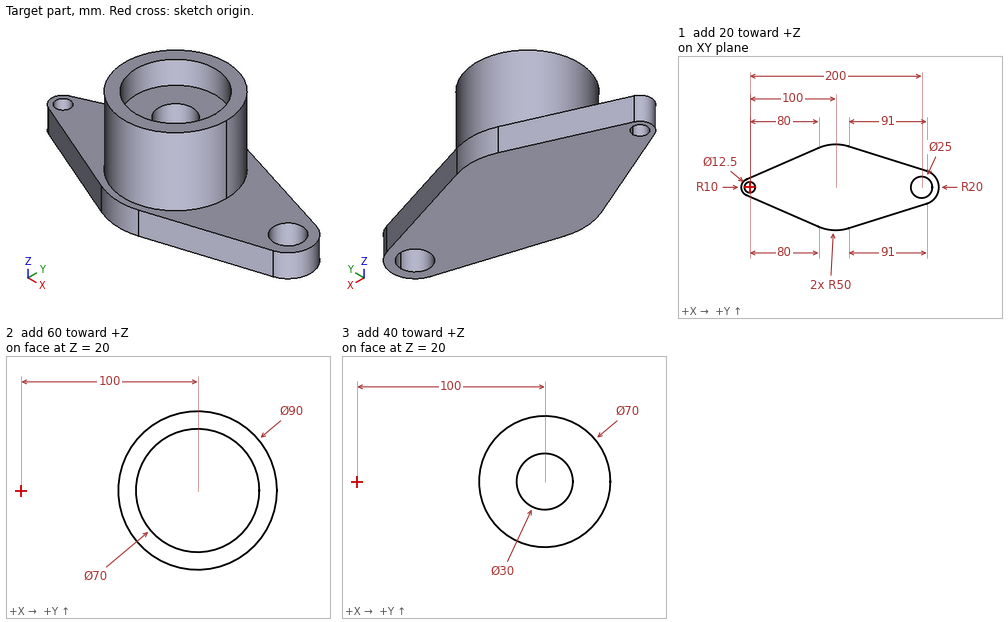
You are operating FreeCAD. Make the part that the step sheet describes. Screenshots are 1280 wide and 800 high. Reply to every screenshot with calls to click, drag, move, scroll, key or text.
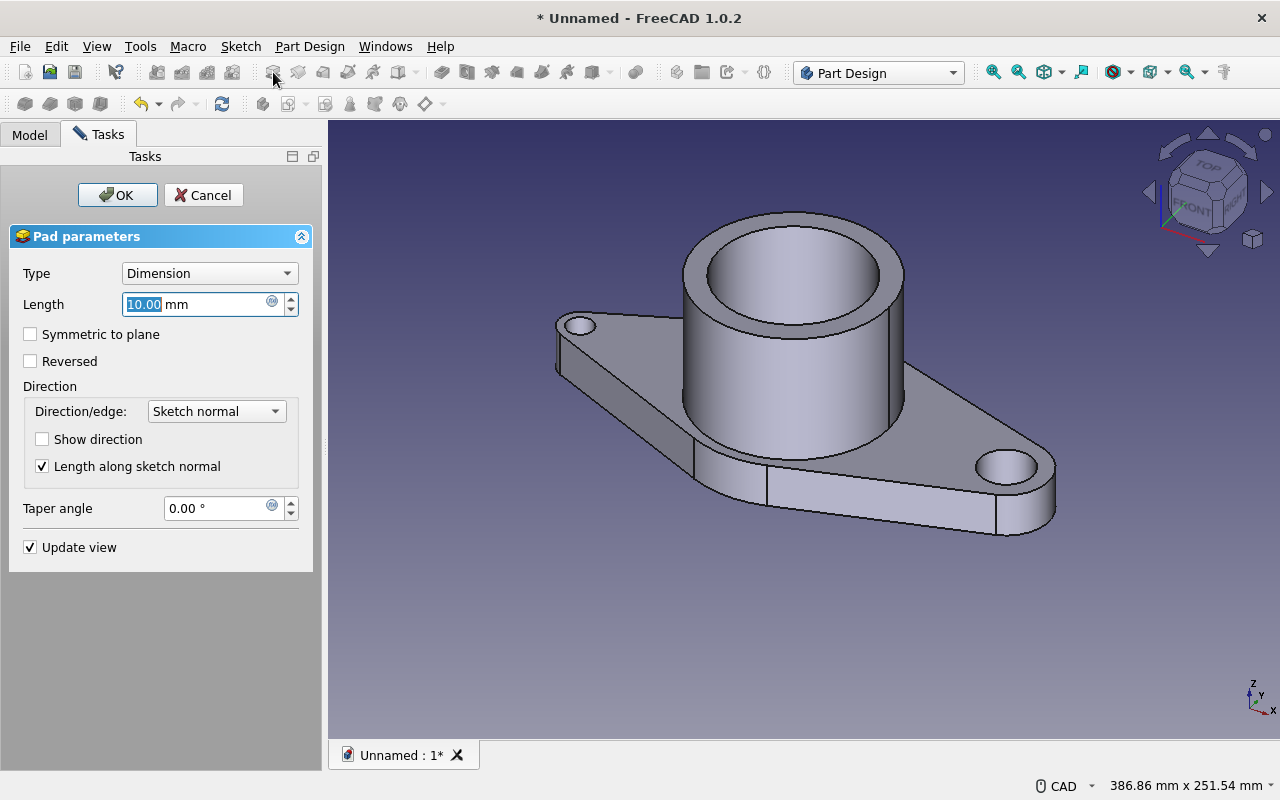
text(40)
key(Tab)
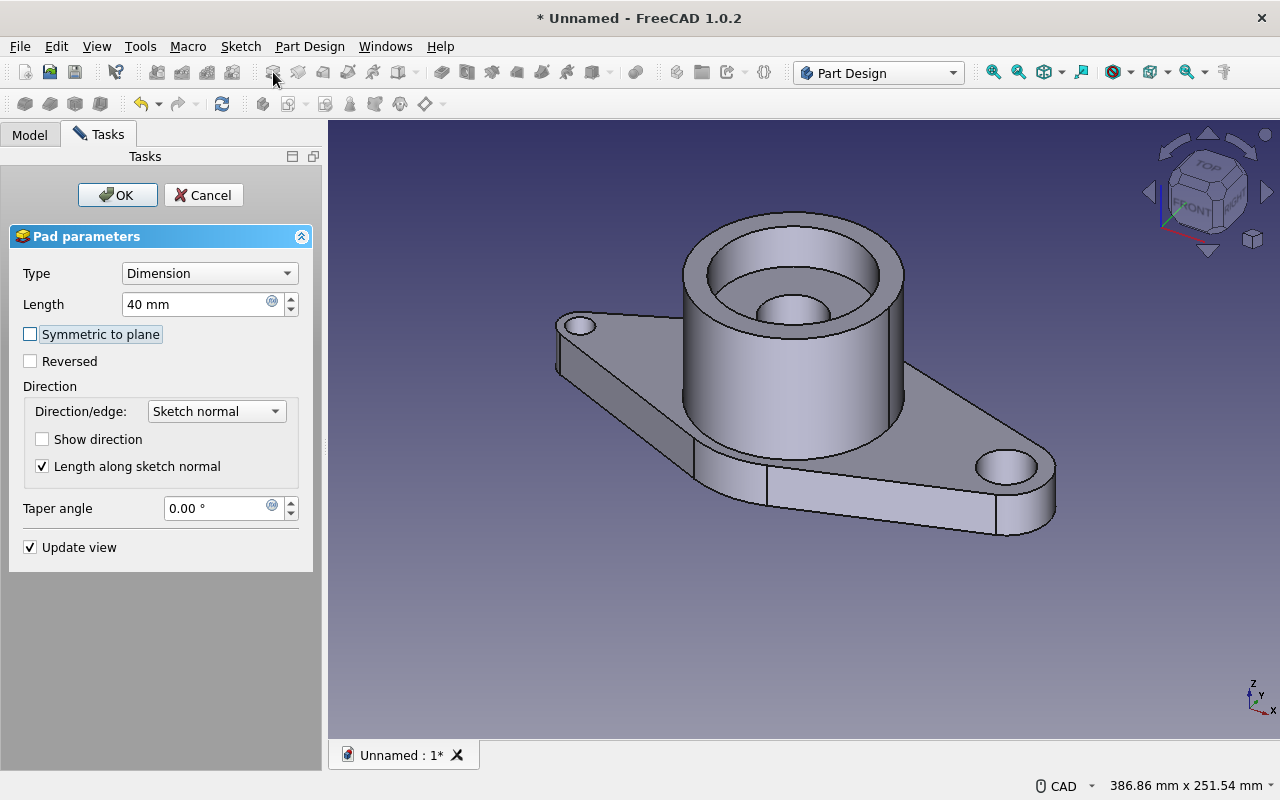
click(118, 195)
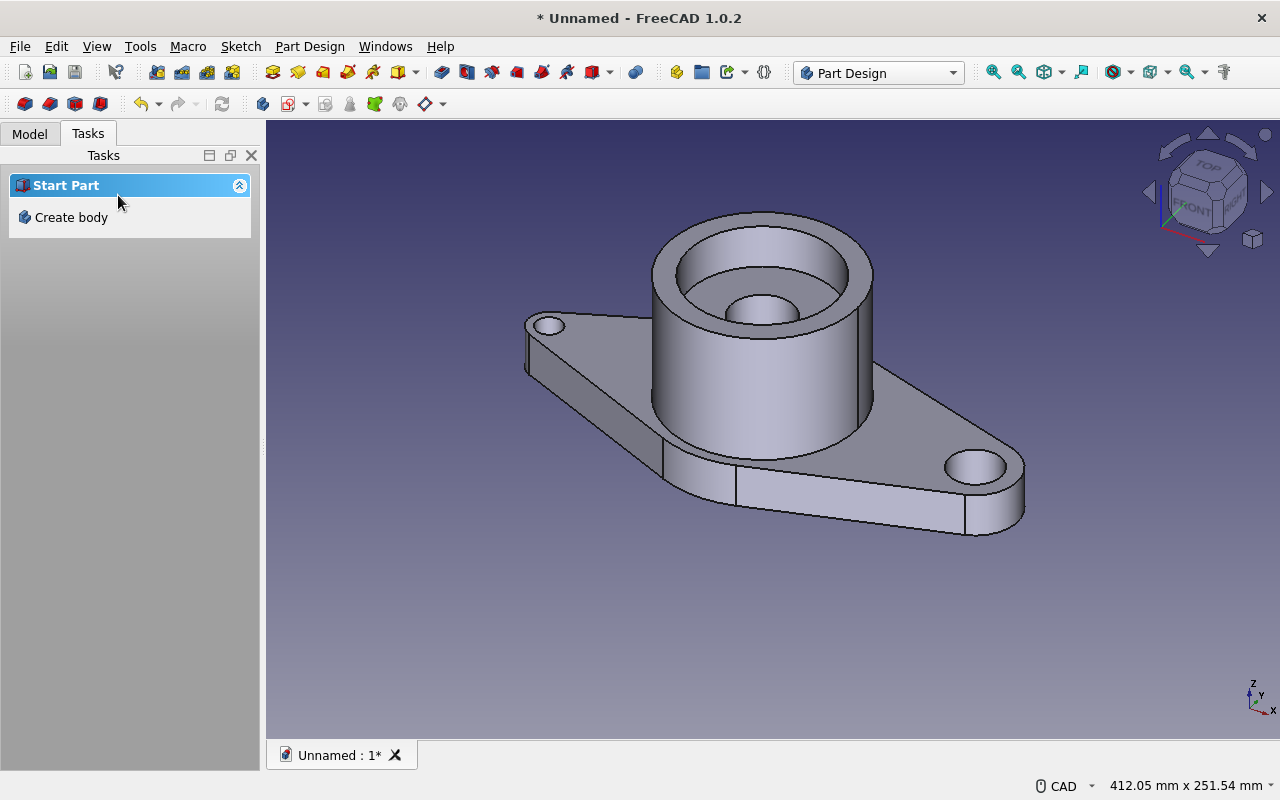
key(0)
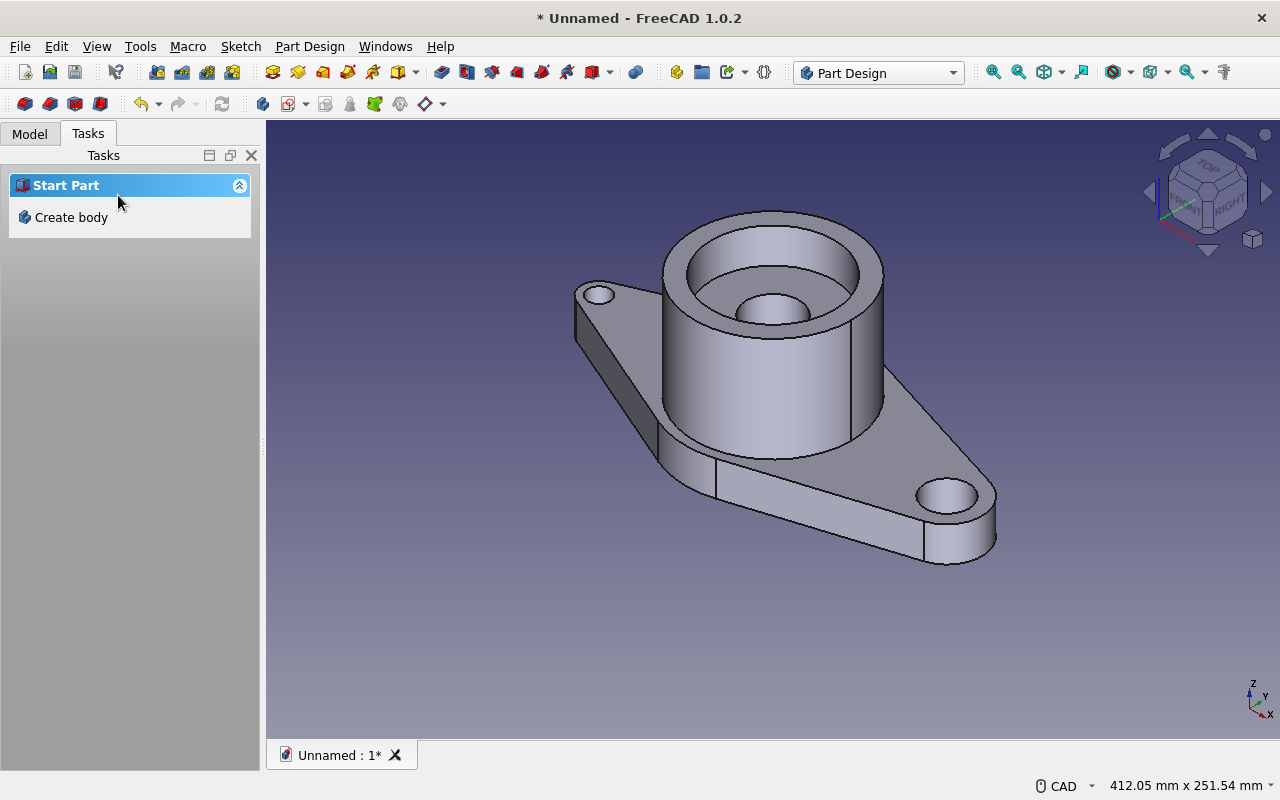
click(994, 72)